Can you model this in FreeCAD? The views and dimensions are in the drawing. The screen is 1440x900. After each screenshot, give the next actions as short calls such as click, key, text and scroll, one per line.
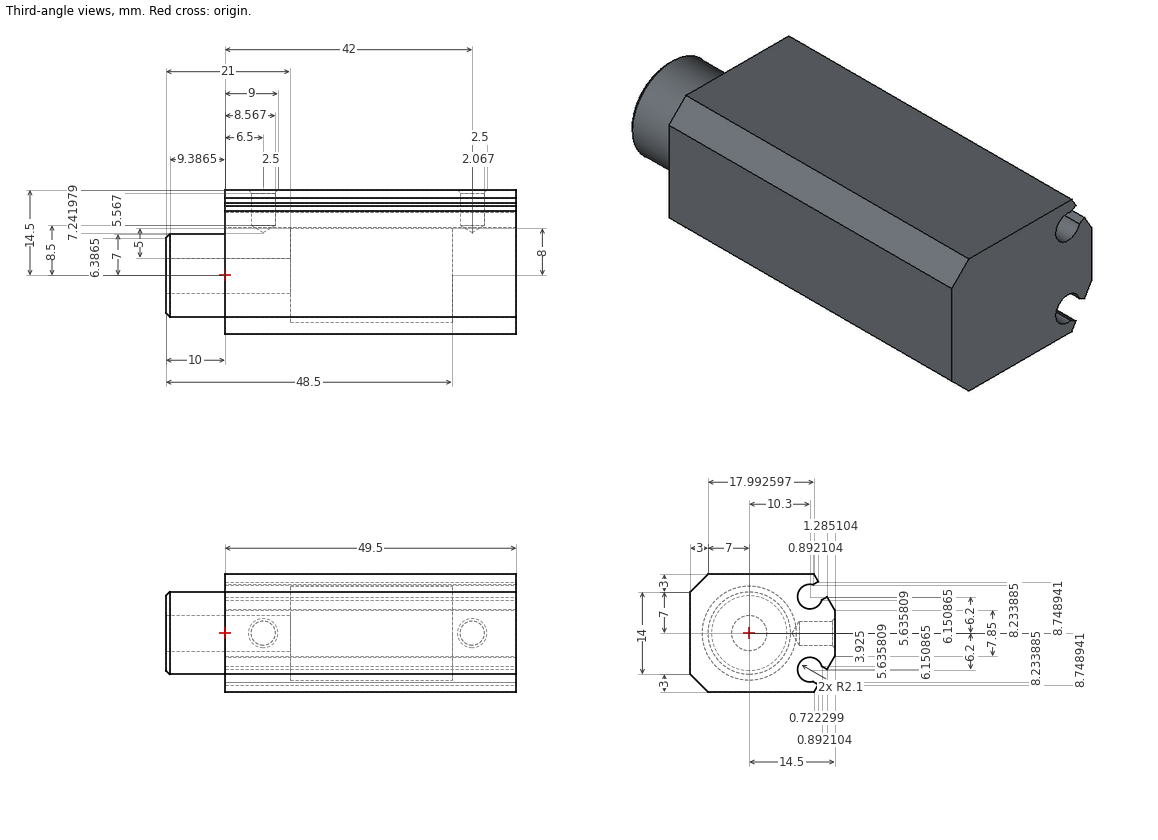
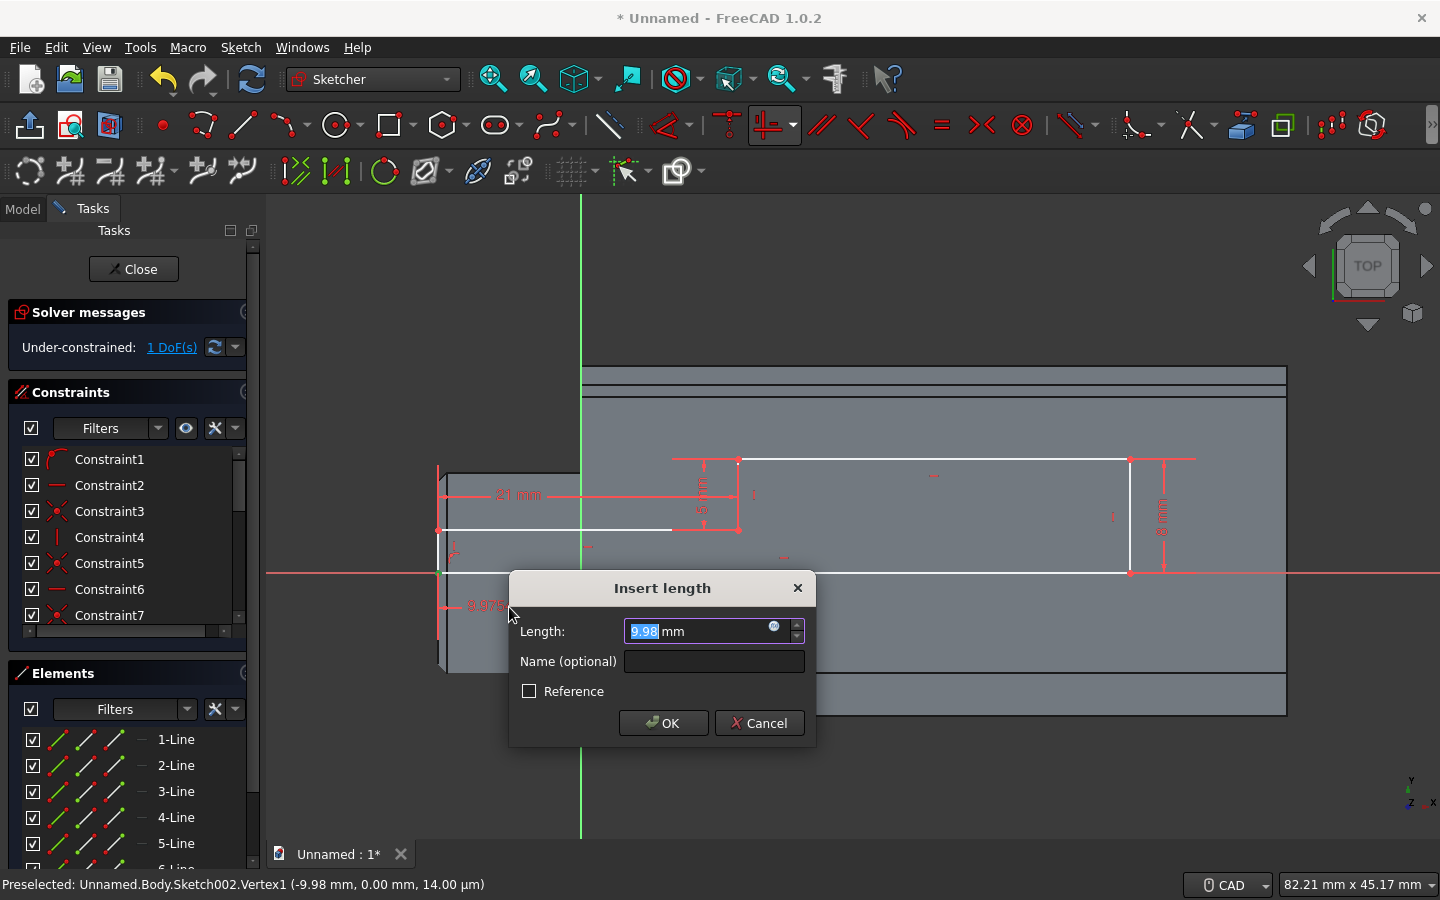
text(10)
key(Return)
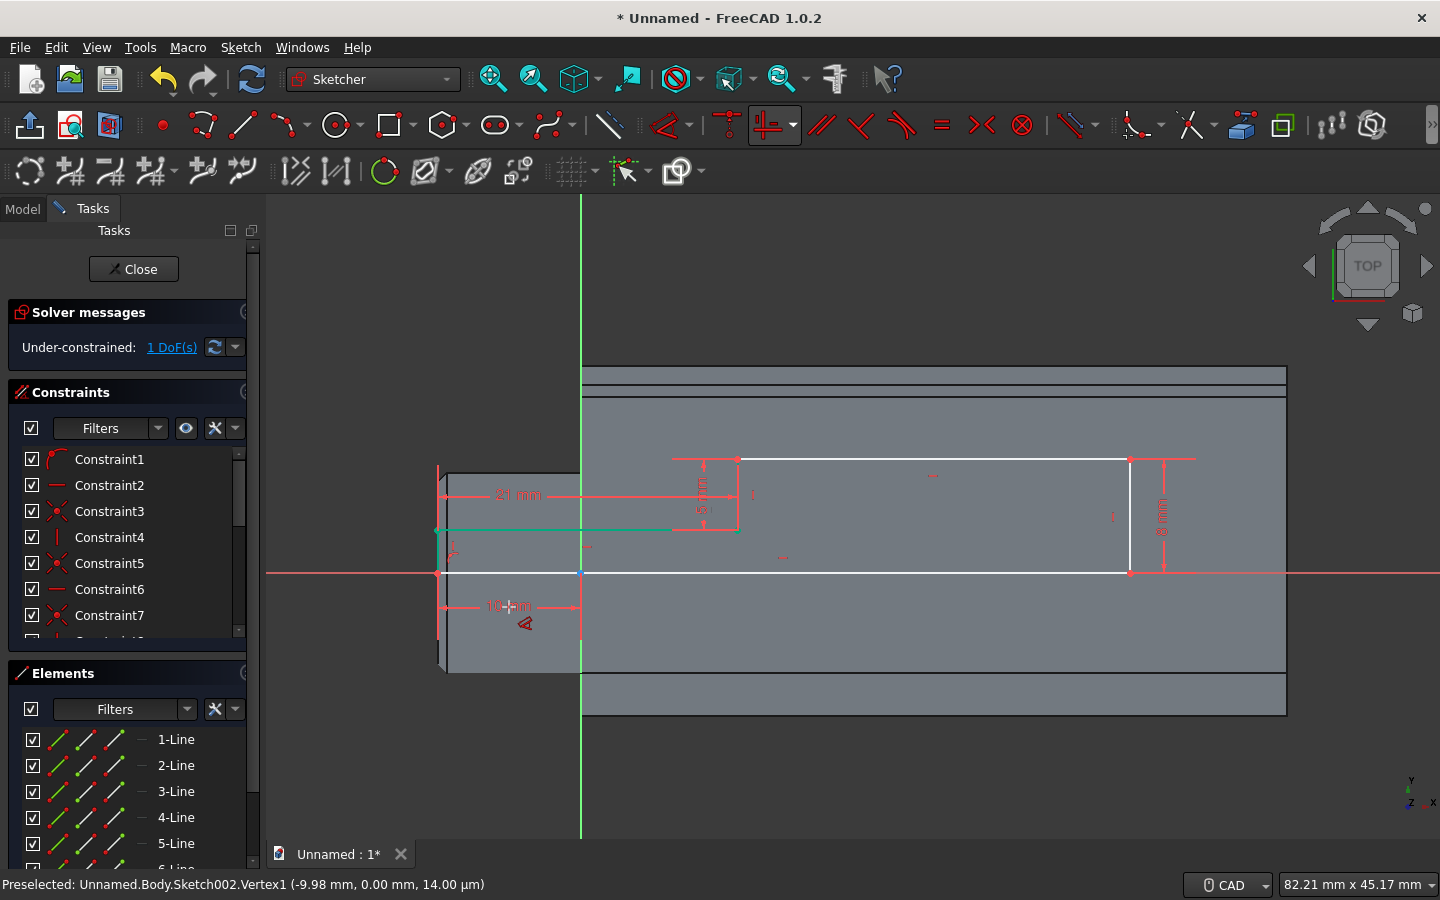
click(645, 573)
click(784, 607)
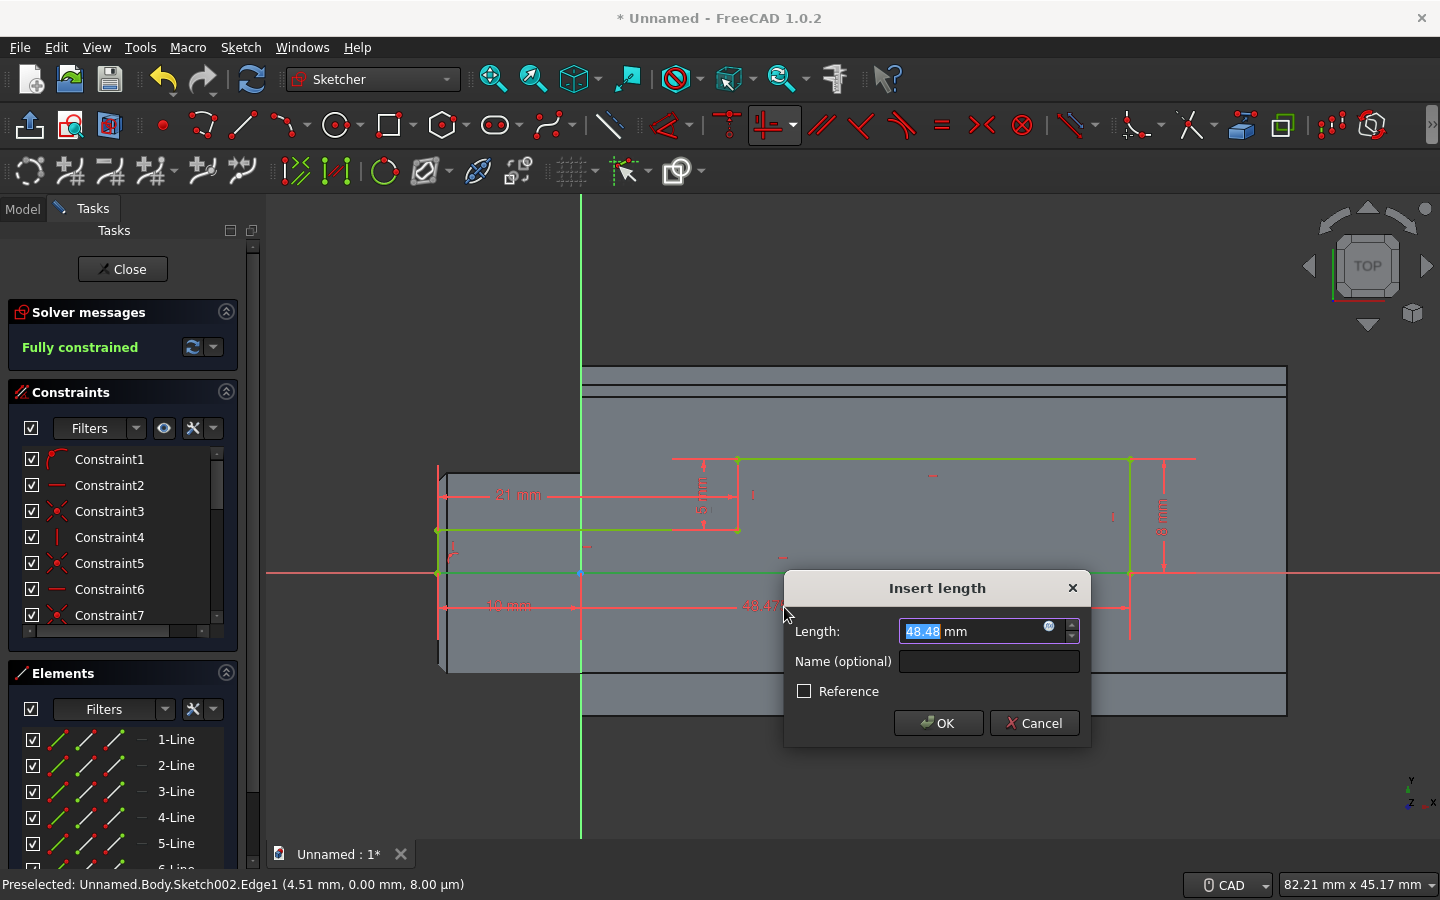
text(48.5)
key(Return)
key(Escape)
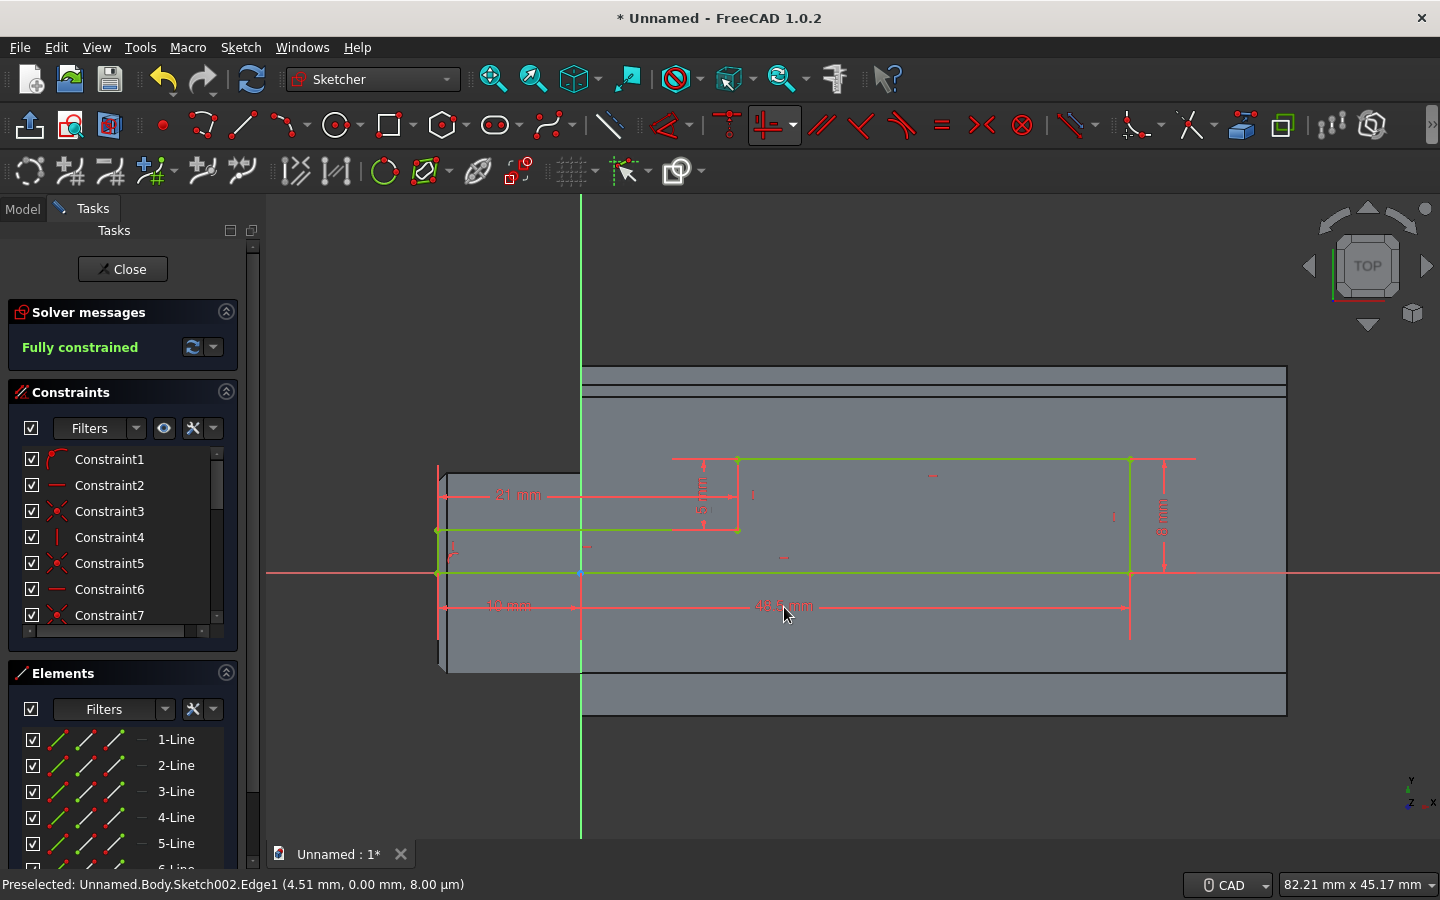
click(123, 269)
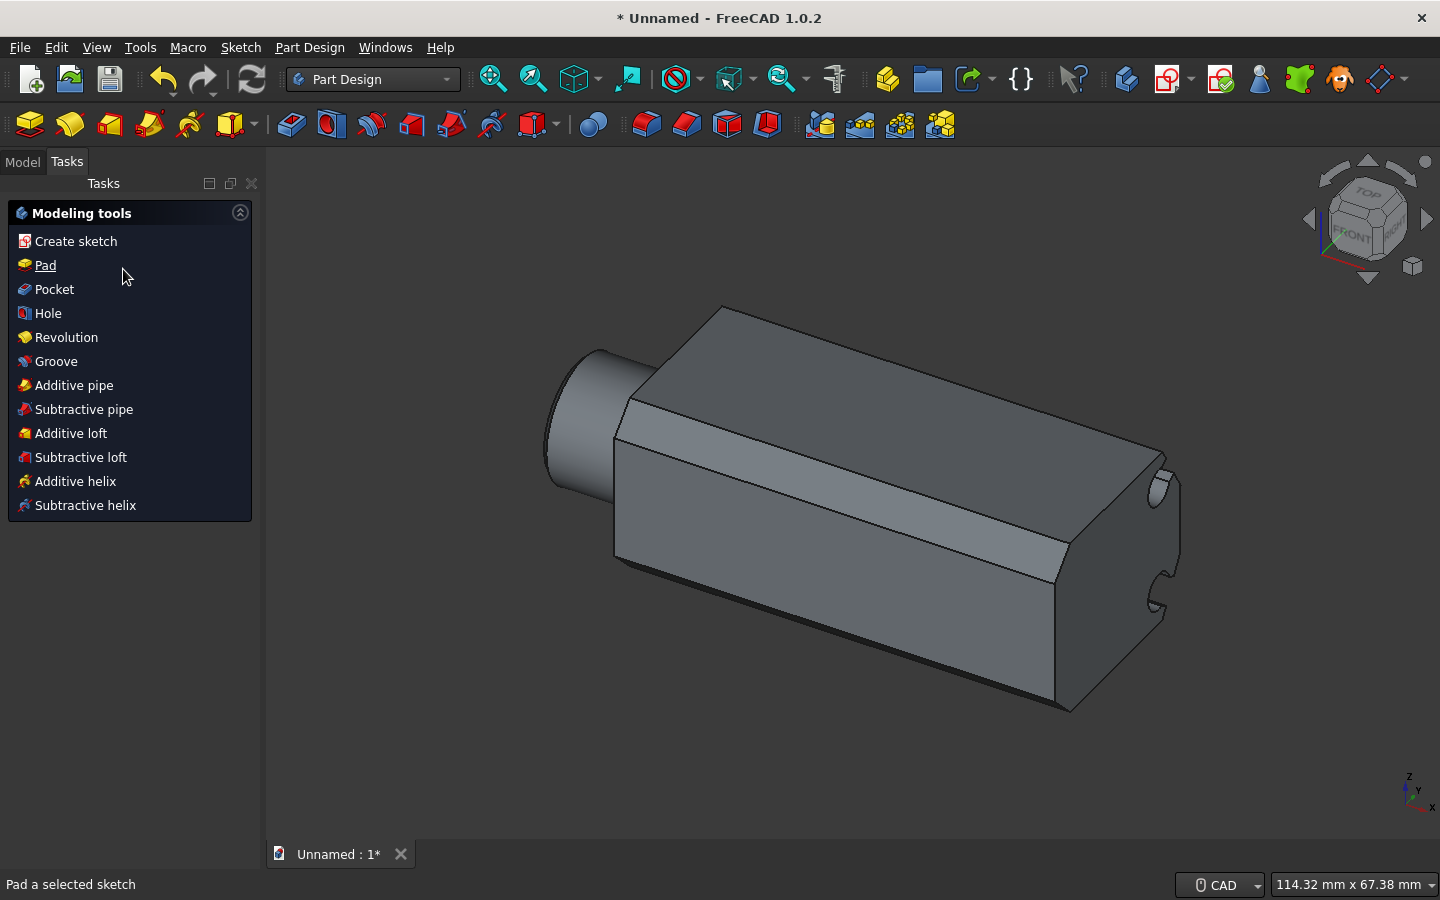
click(372, 124)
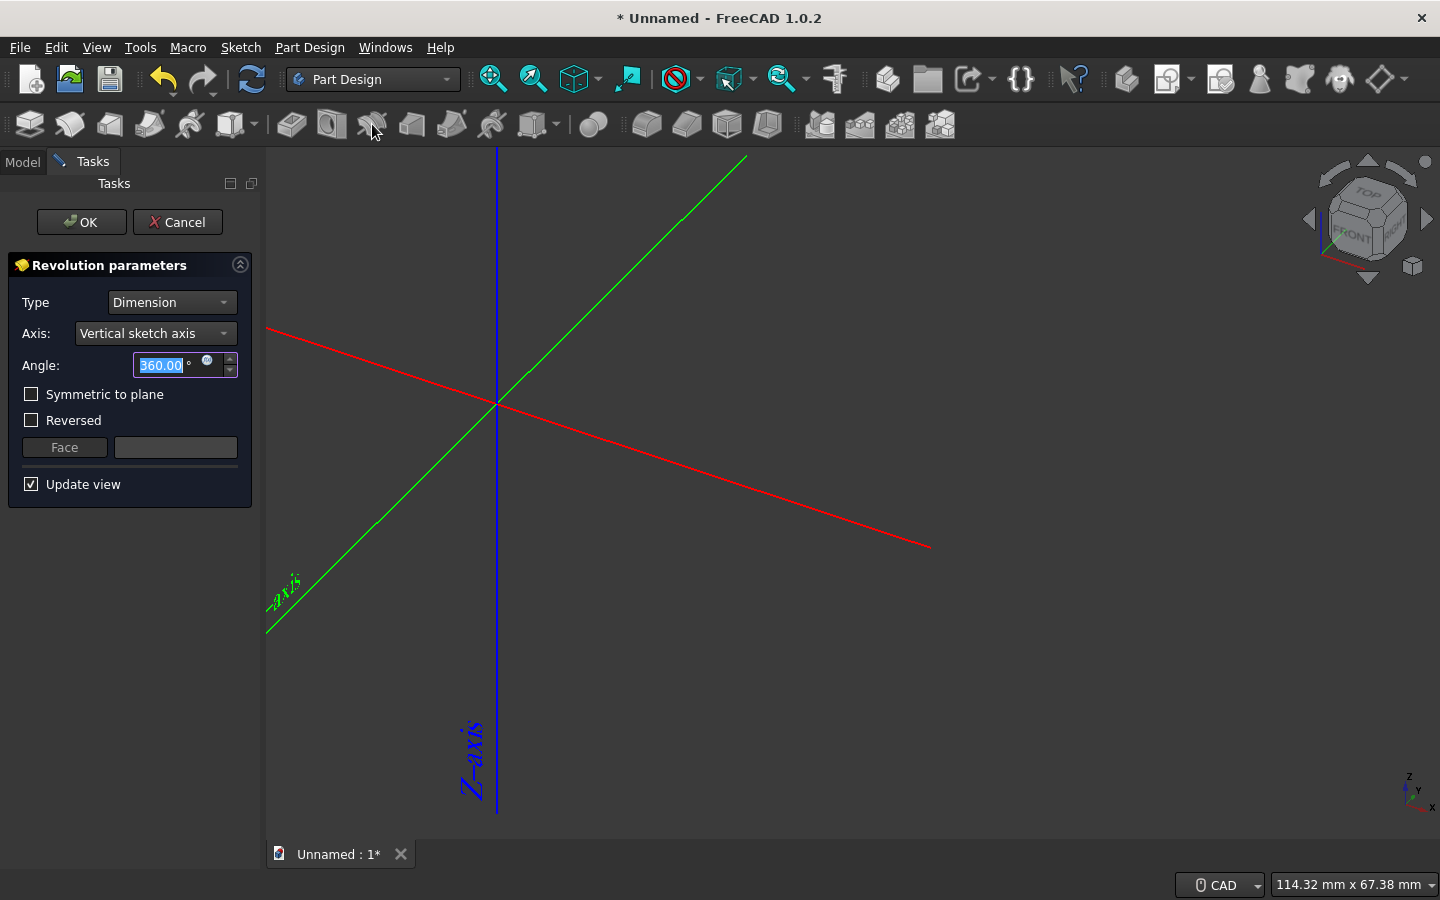
click(156, 334)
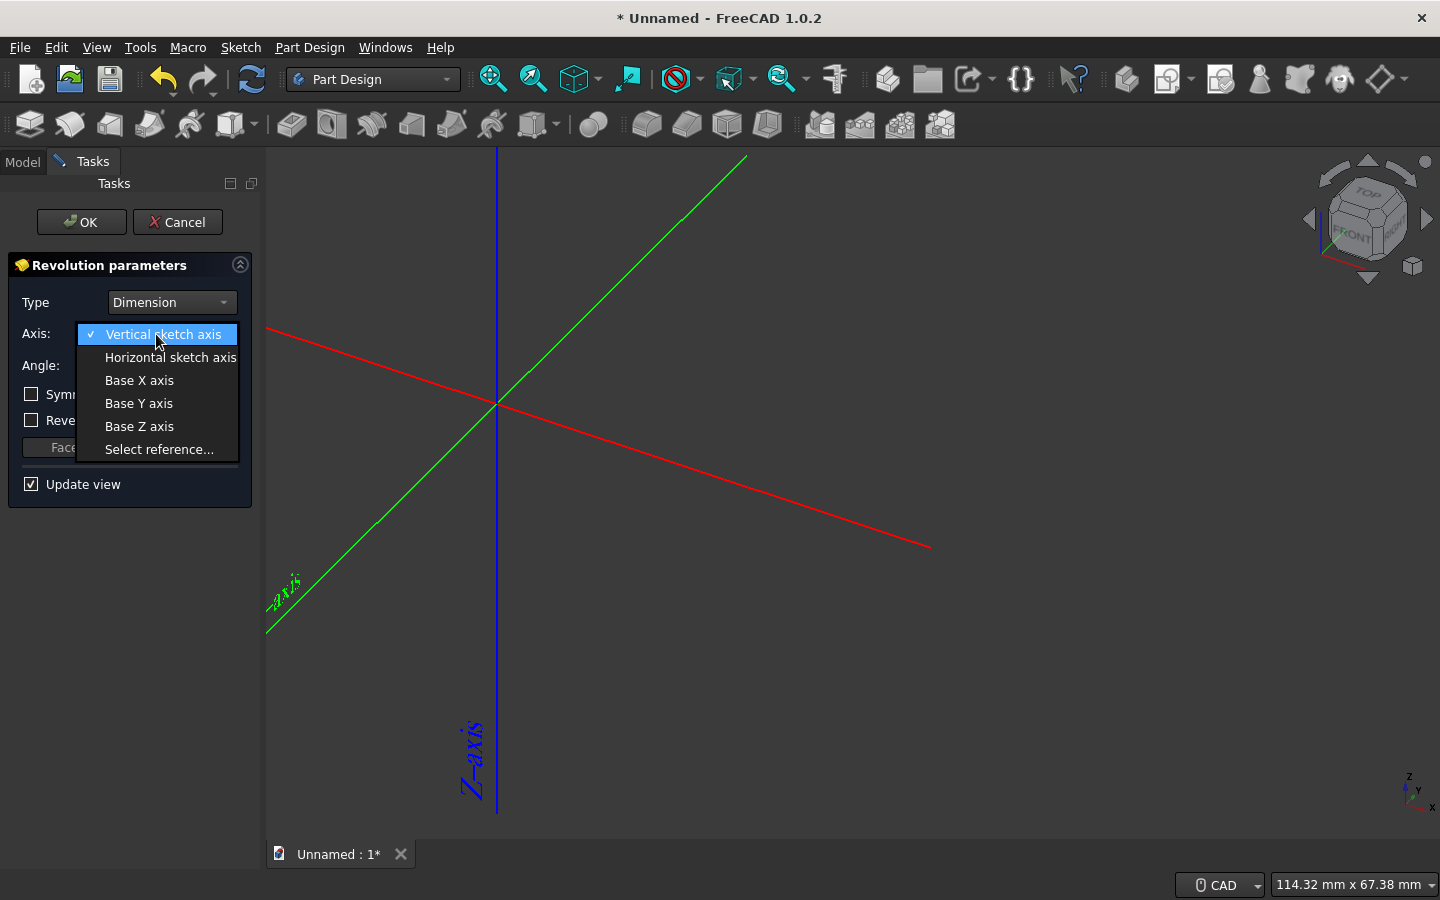
click(156, 358)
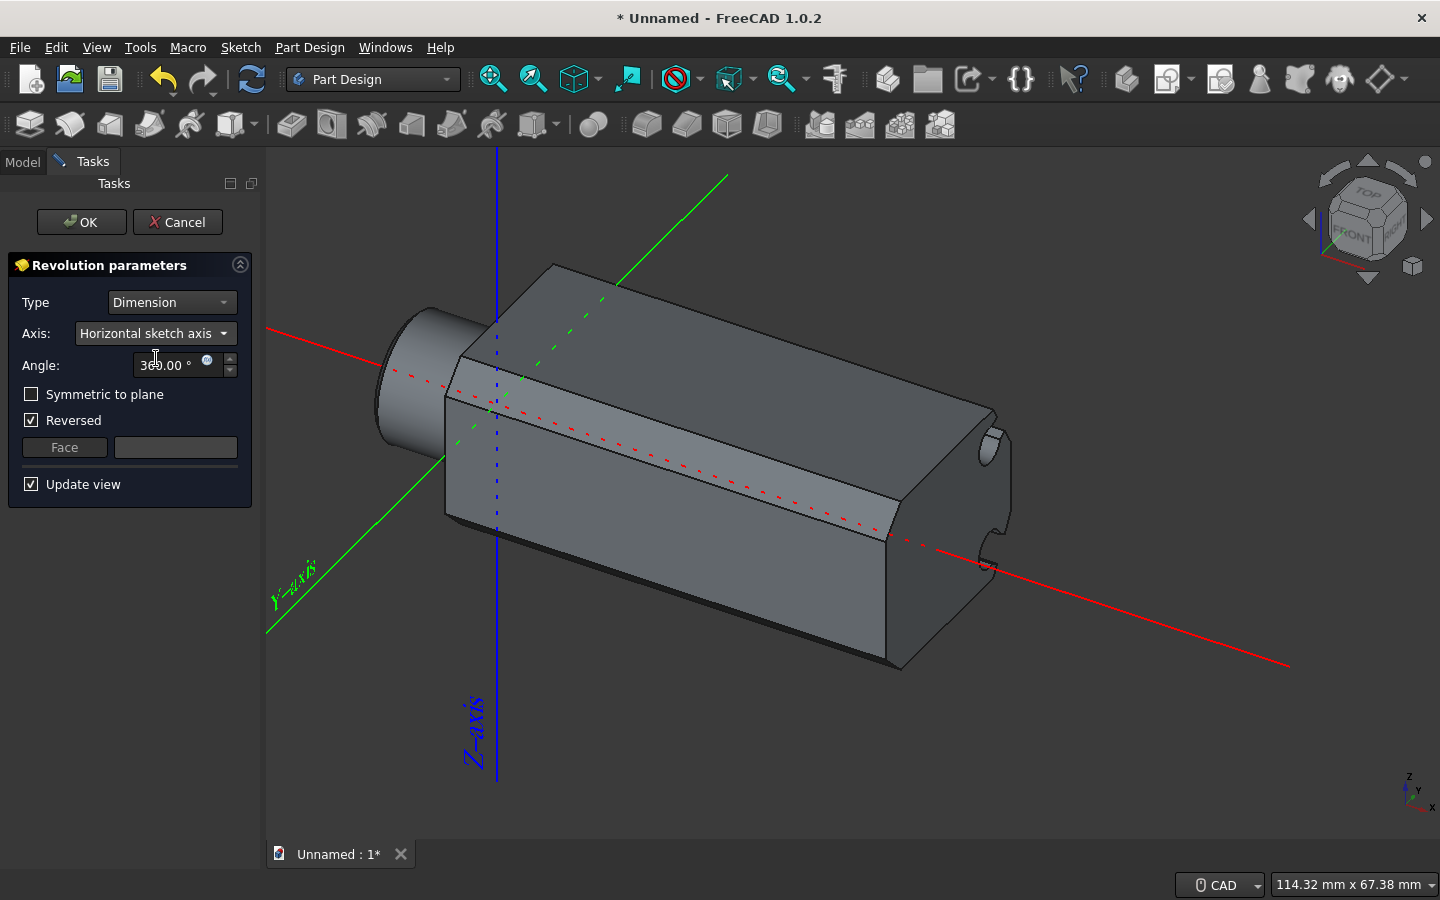
click(82, 222)